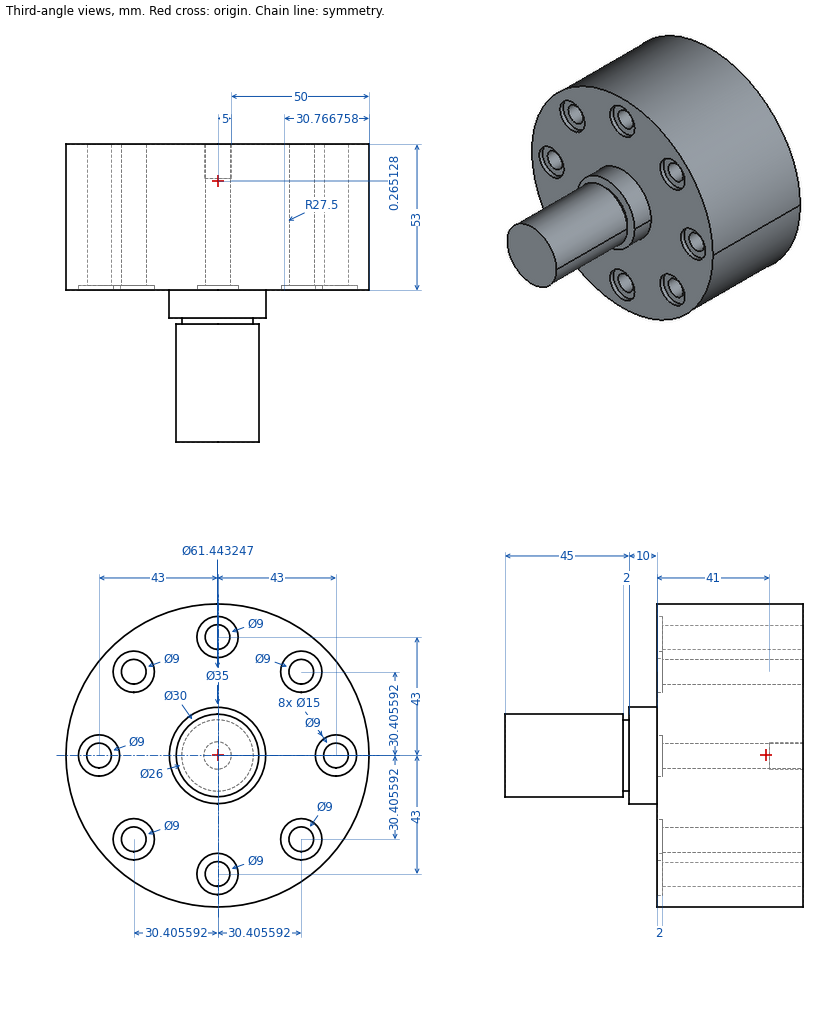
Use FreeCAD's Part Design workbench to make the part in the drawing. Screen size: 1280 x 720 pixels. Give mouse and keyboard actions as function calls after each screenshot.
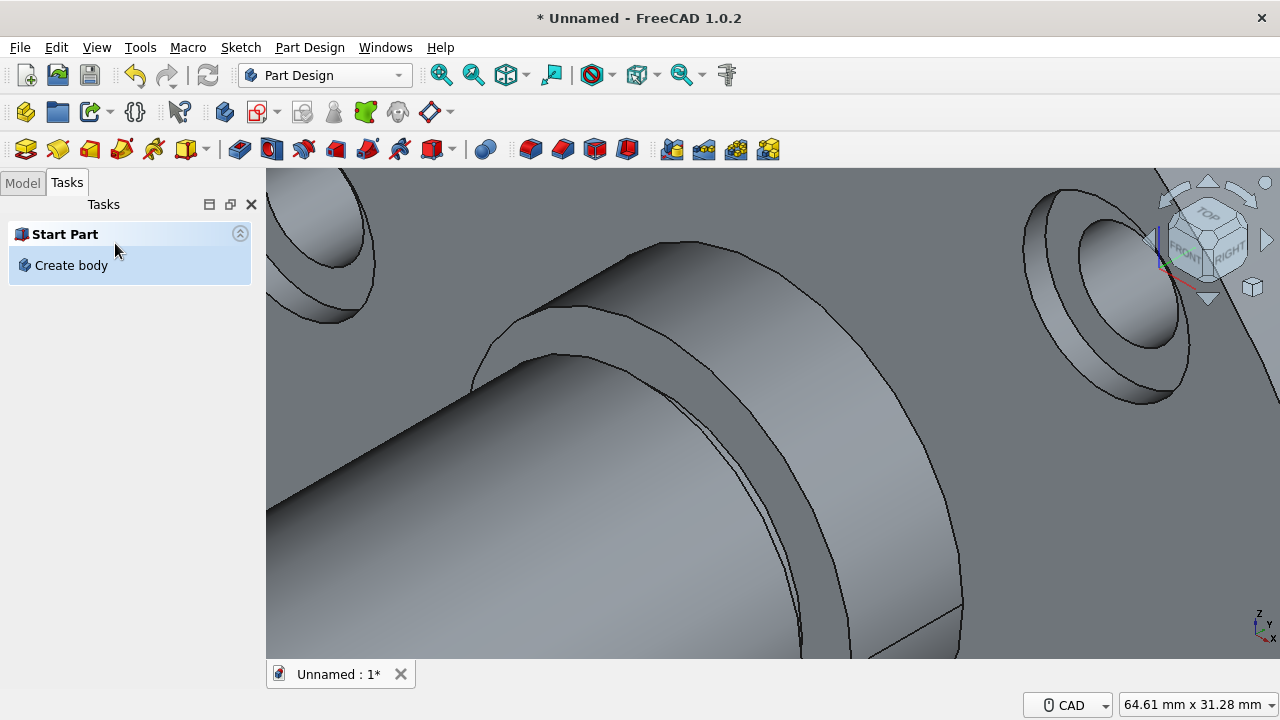
key(v)
key(f)